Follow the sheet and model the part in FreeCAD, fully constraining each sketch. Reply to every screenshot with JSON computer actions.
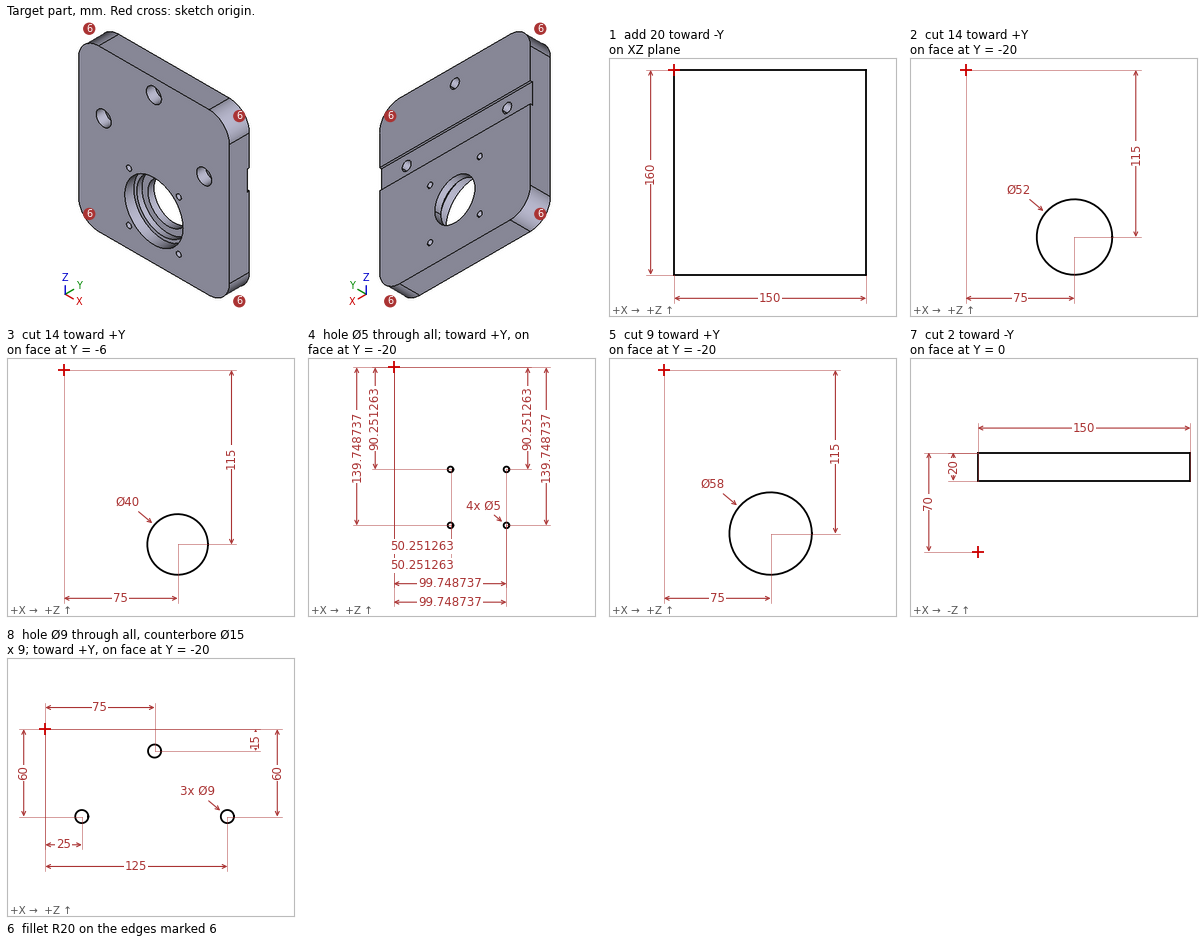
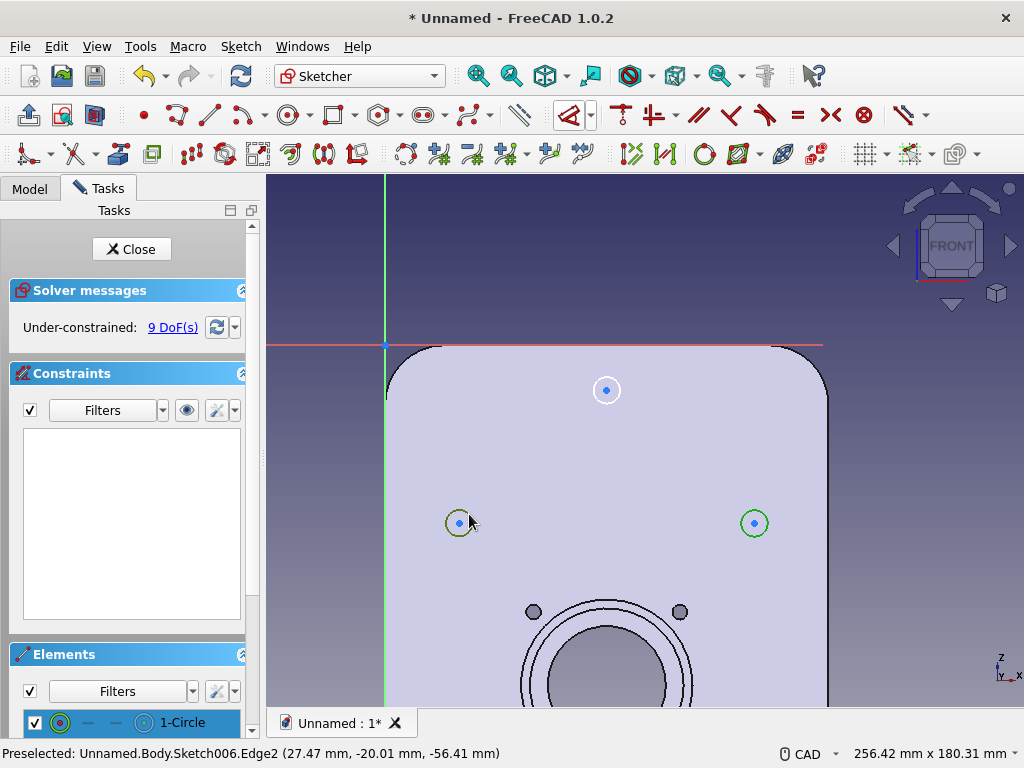
{"action": "left_click", "coordinate": [616, 381]}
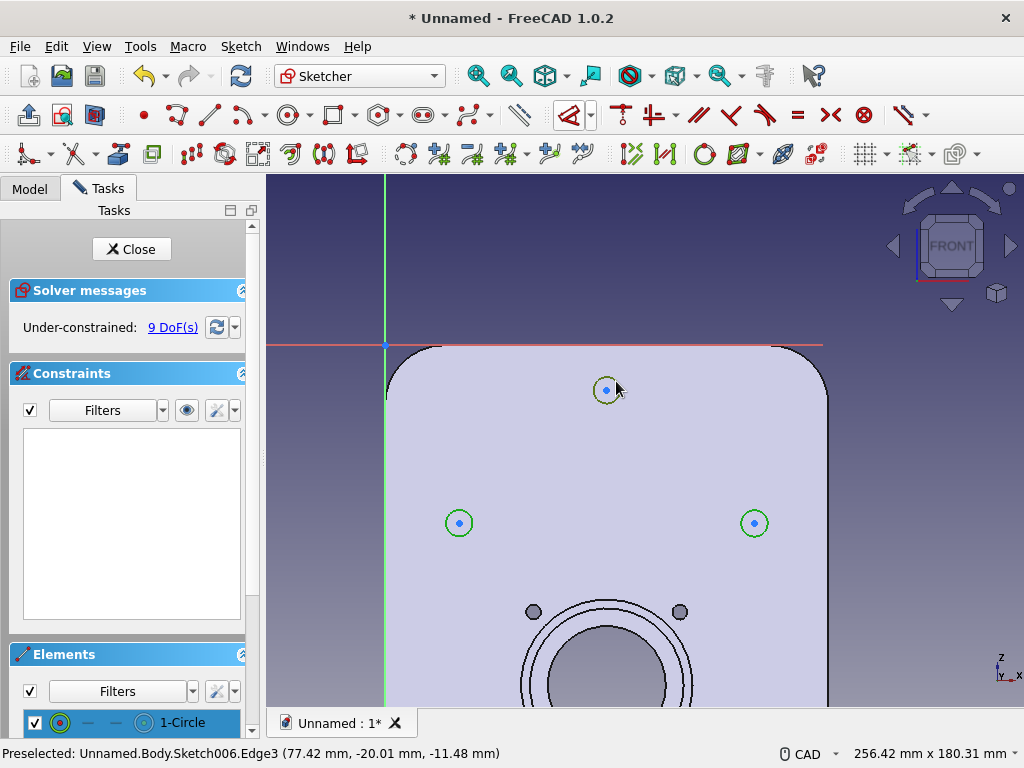
{"action": "left_click", "coordinate": [798, 116]}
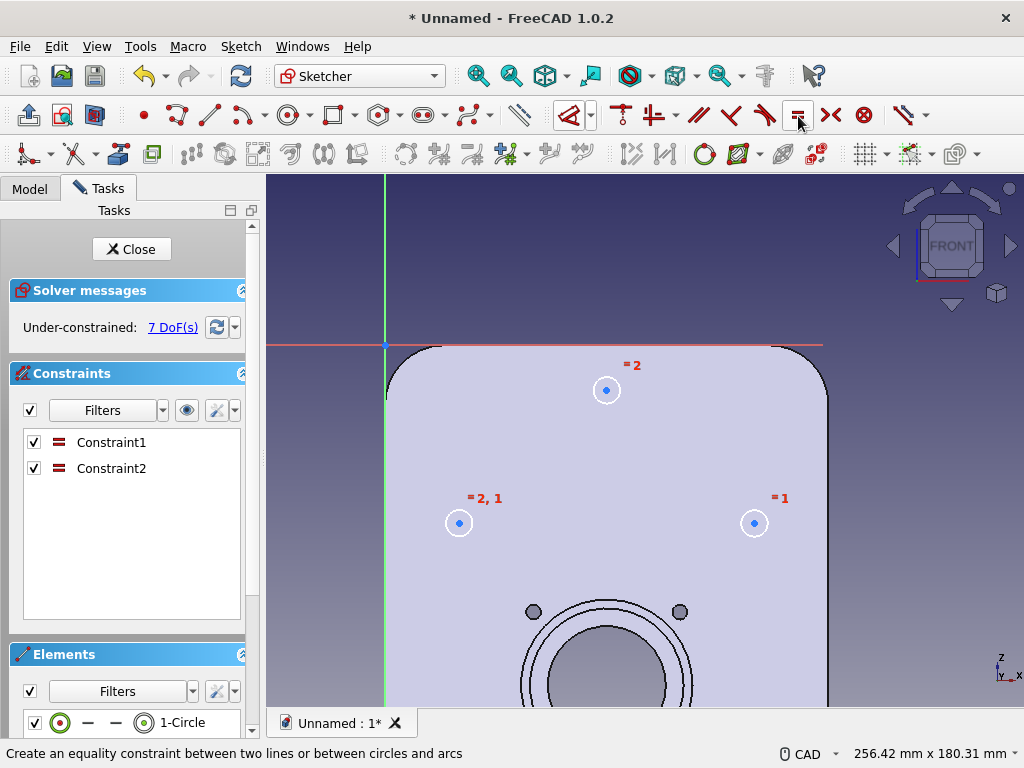
{"action": "scroll", "coordinate": [764, 514], "scroll_direction": "up", "scroll_amount": 3}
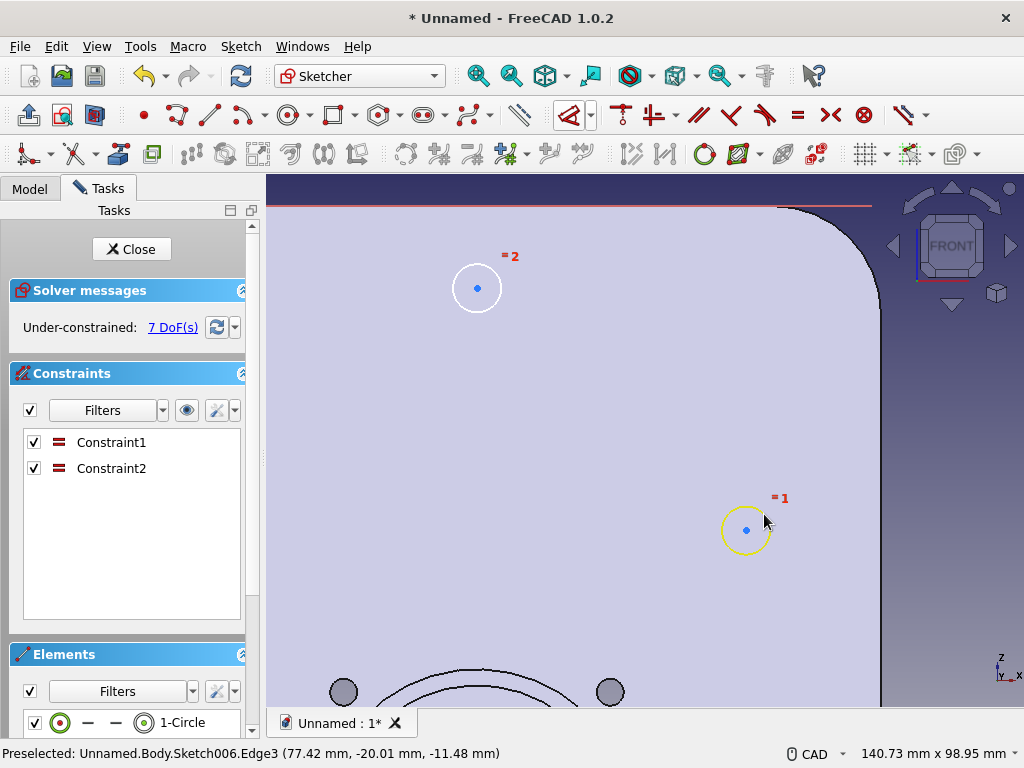
{"action": "left_click", "coordinate": [763, 513]}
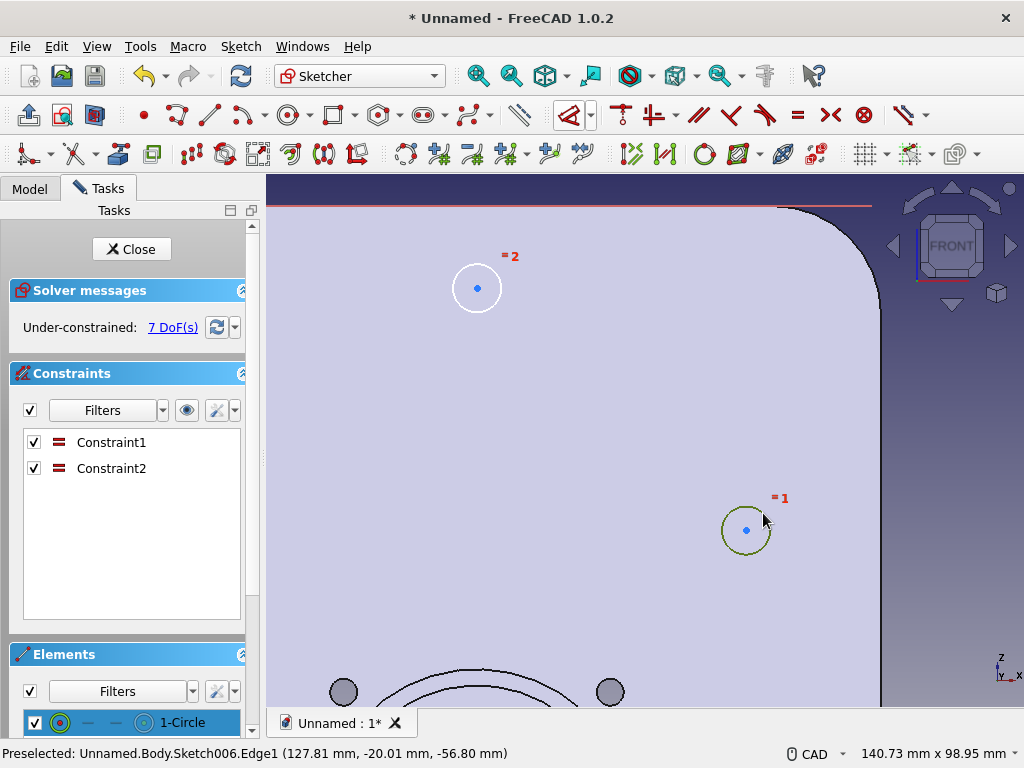
{"action": "key", "text": "k o"}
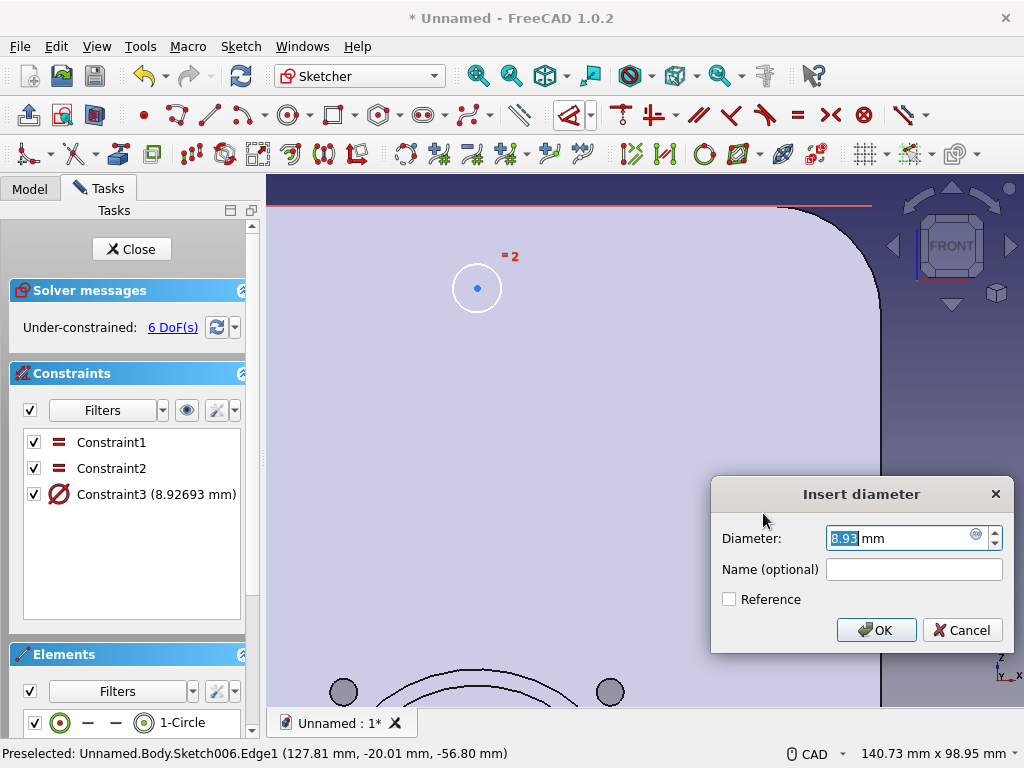
{"action": "type", "text": "9"}
{"action": "key", "text": "Return"}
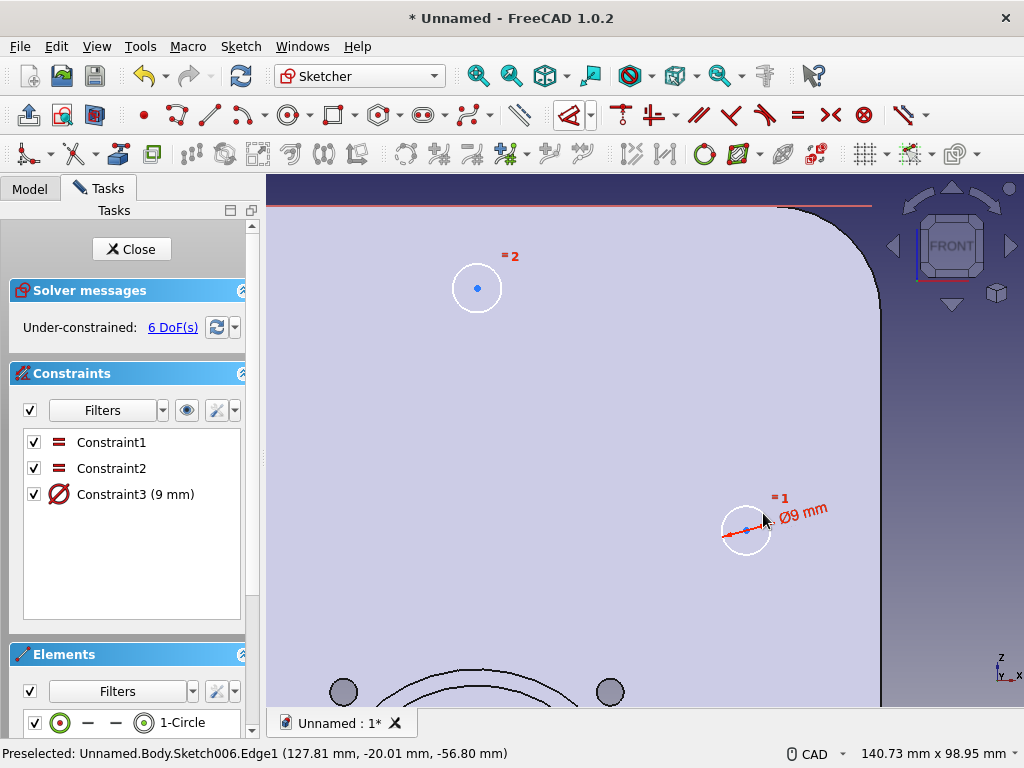
{"action": "left_click", "coordinate": [746, 531]}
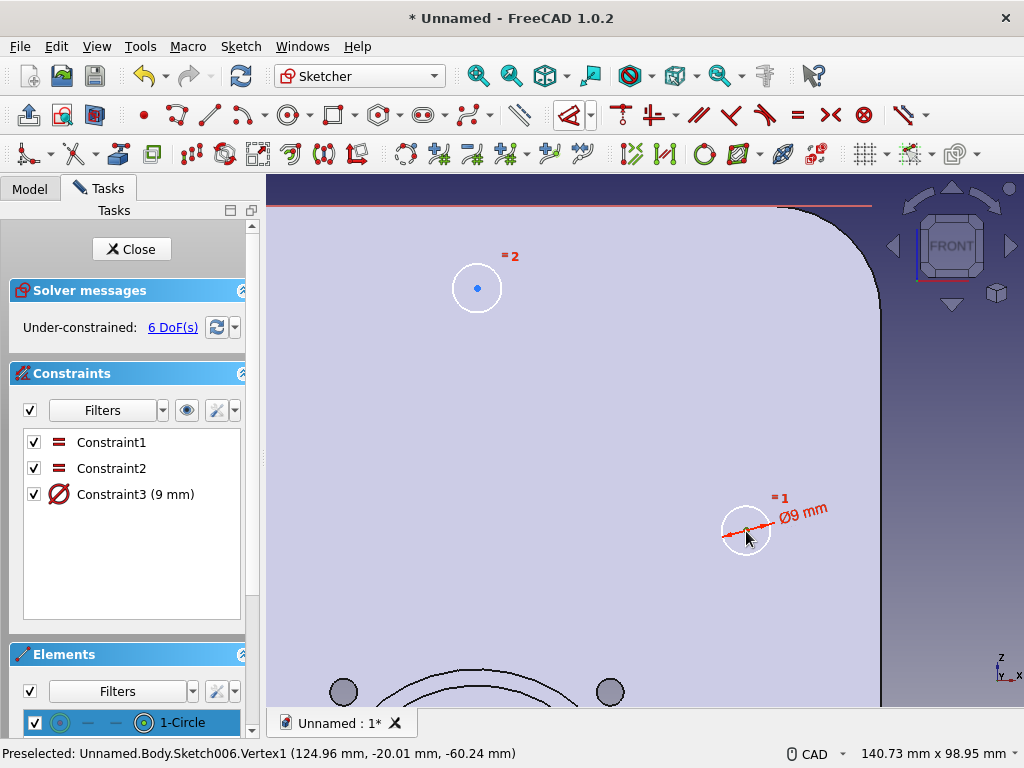
{"action": "left_click", "coordinate": [590, 116]}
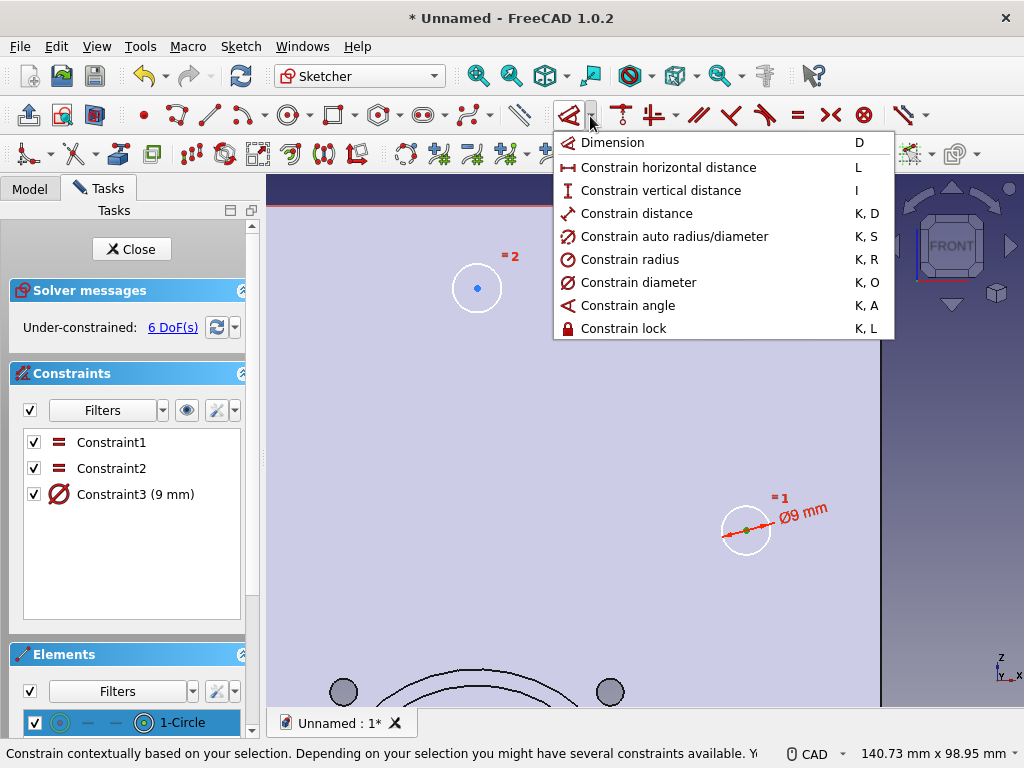
{"action": "left_click", "coordinate": [724, 190]}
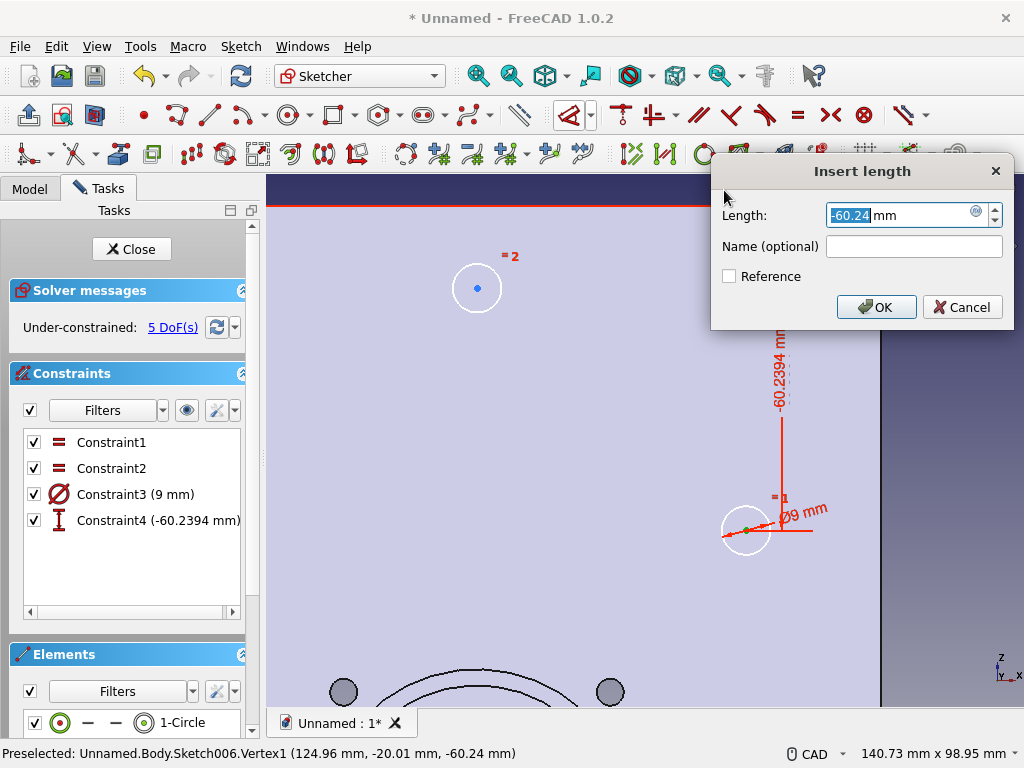
{"action": "type", "text": "-60"}
{"action": "key", "text": "Return"}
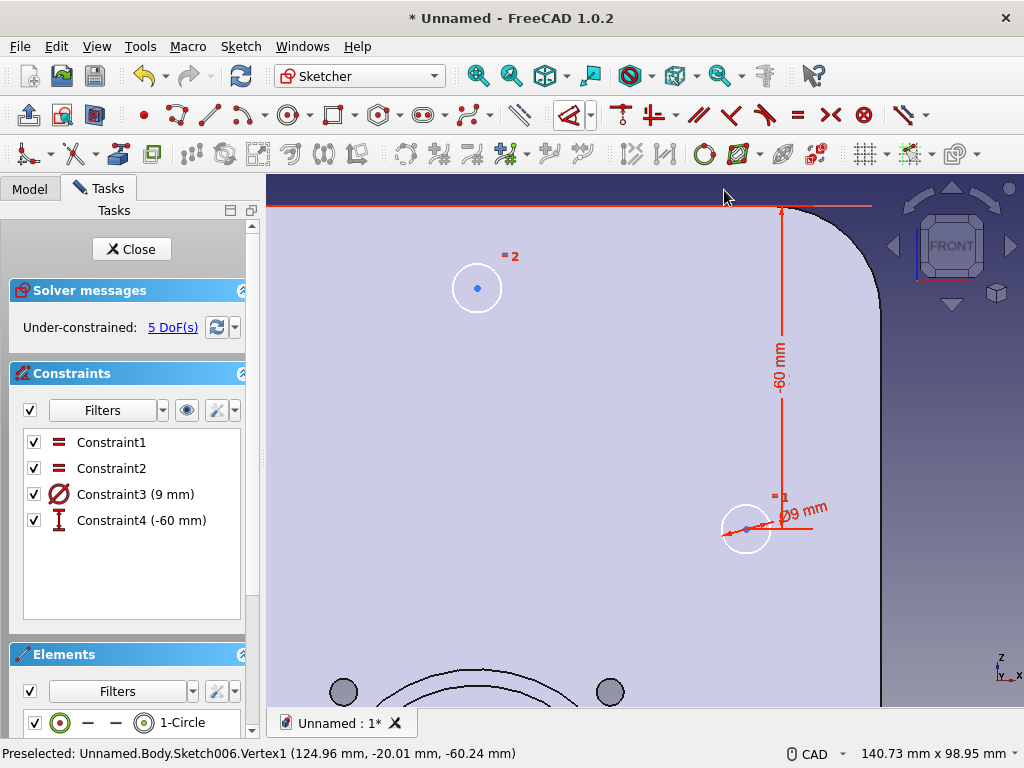
{"action": "scroll", "coordinate": [765, 514], "scroll_direction": "down", "scroll_amount": 3}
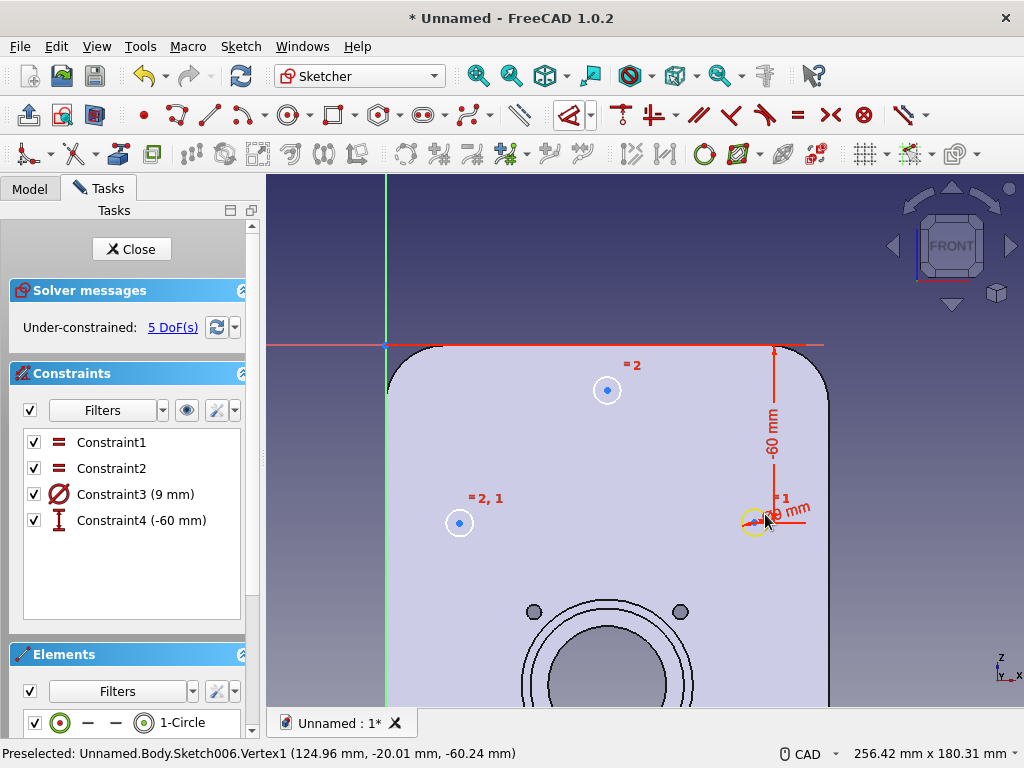
{"action": "left_click", "coordinate": [460, 523]}